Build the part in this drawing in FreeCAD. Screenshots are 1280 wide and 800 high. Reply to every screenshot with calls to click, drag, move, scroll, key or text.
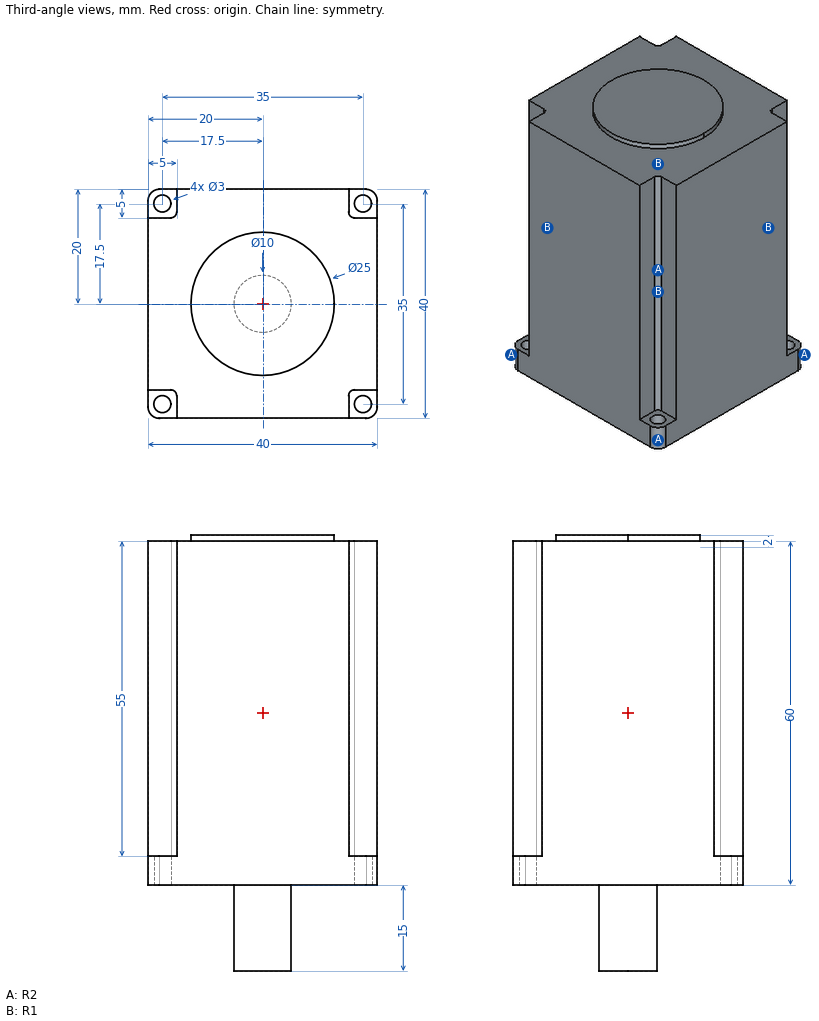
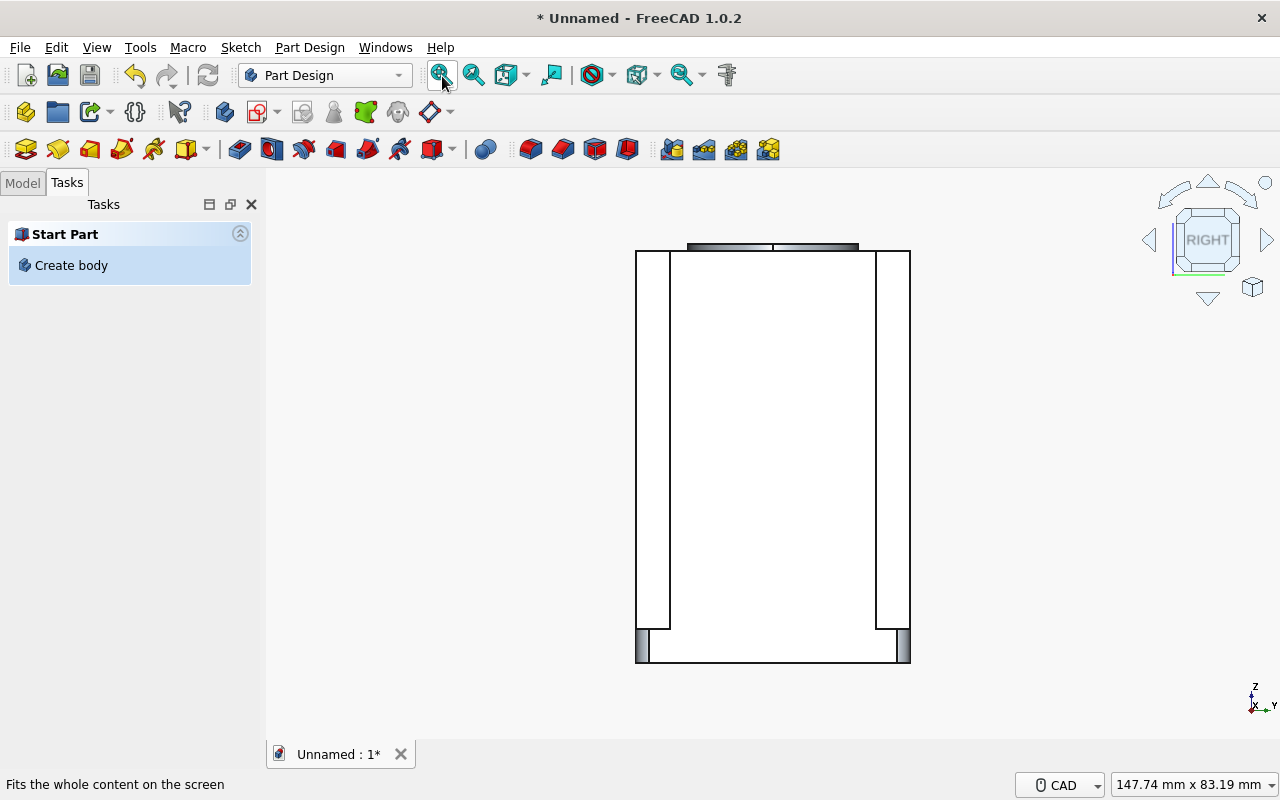
key(5)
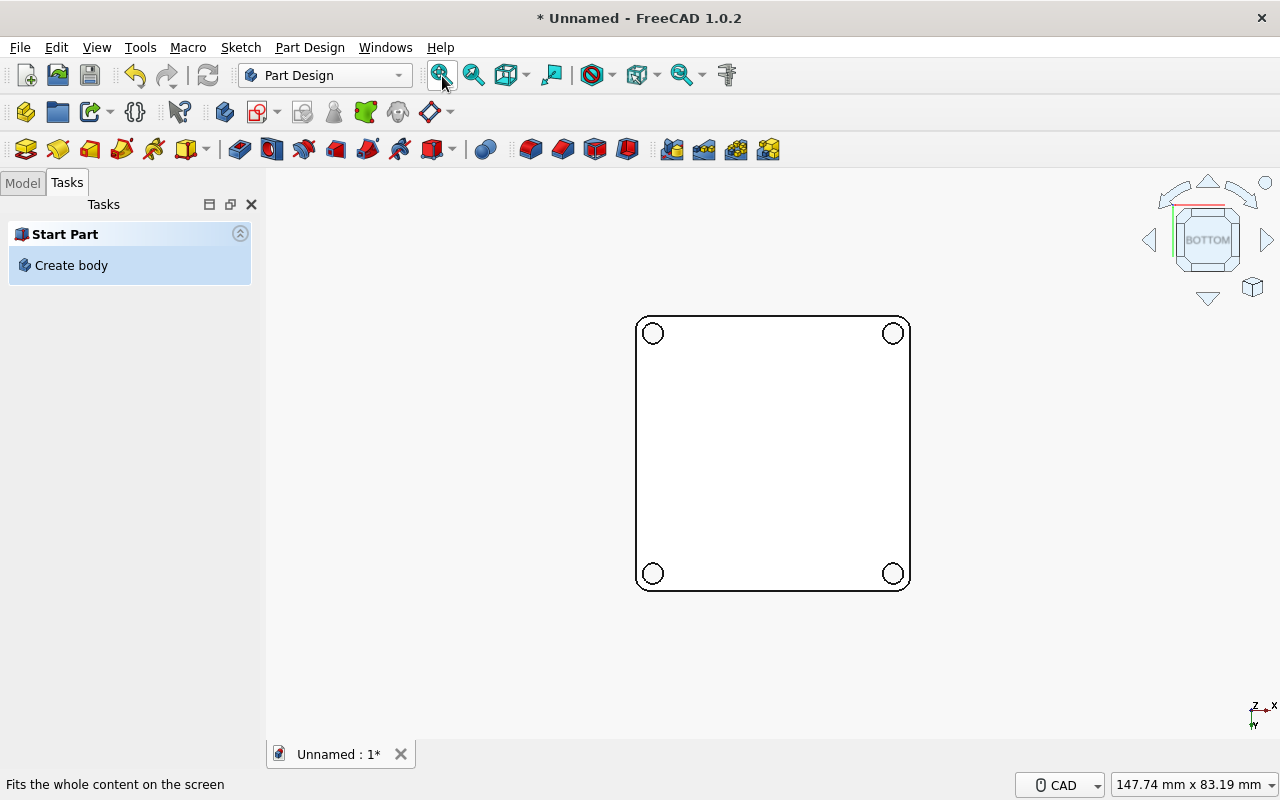
key(4)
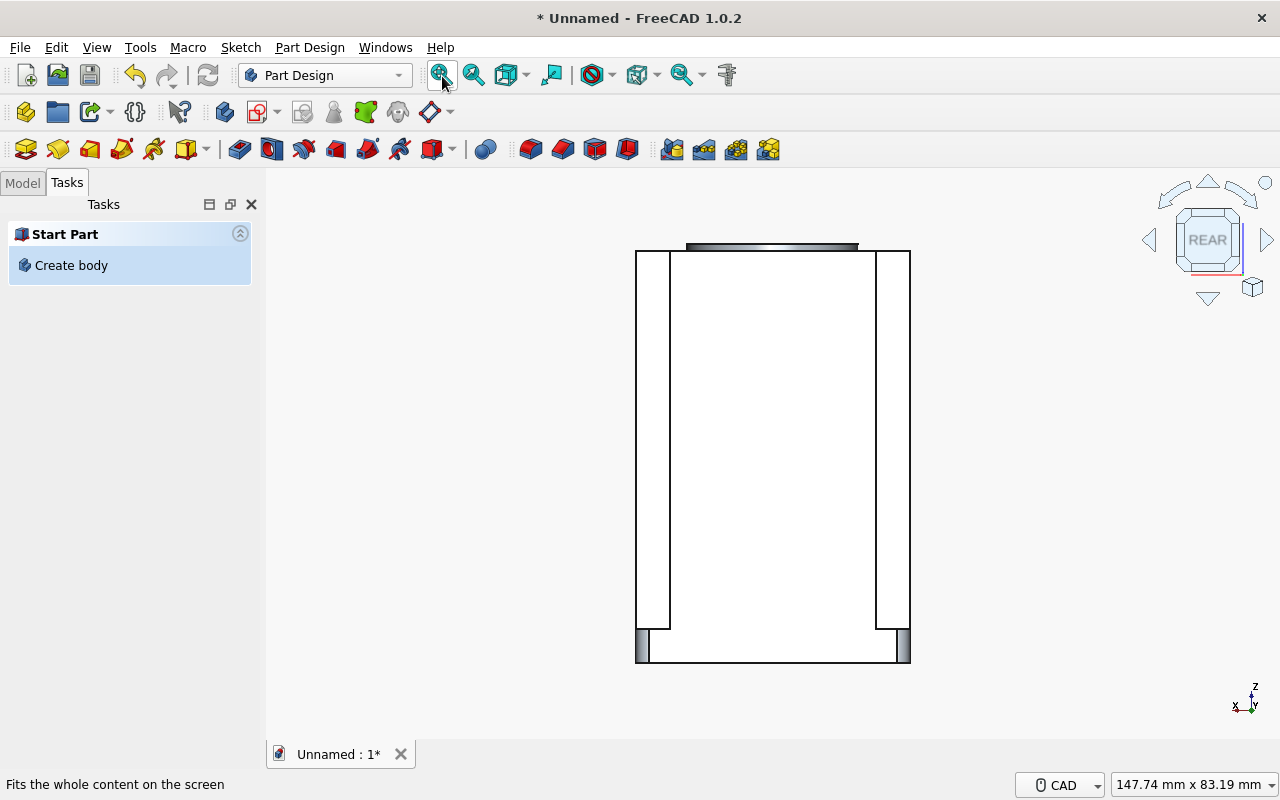
key(6)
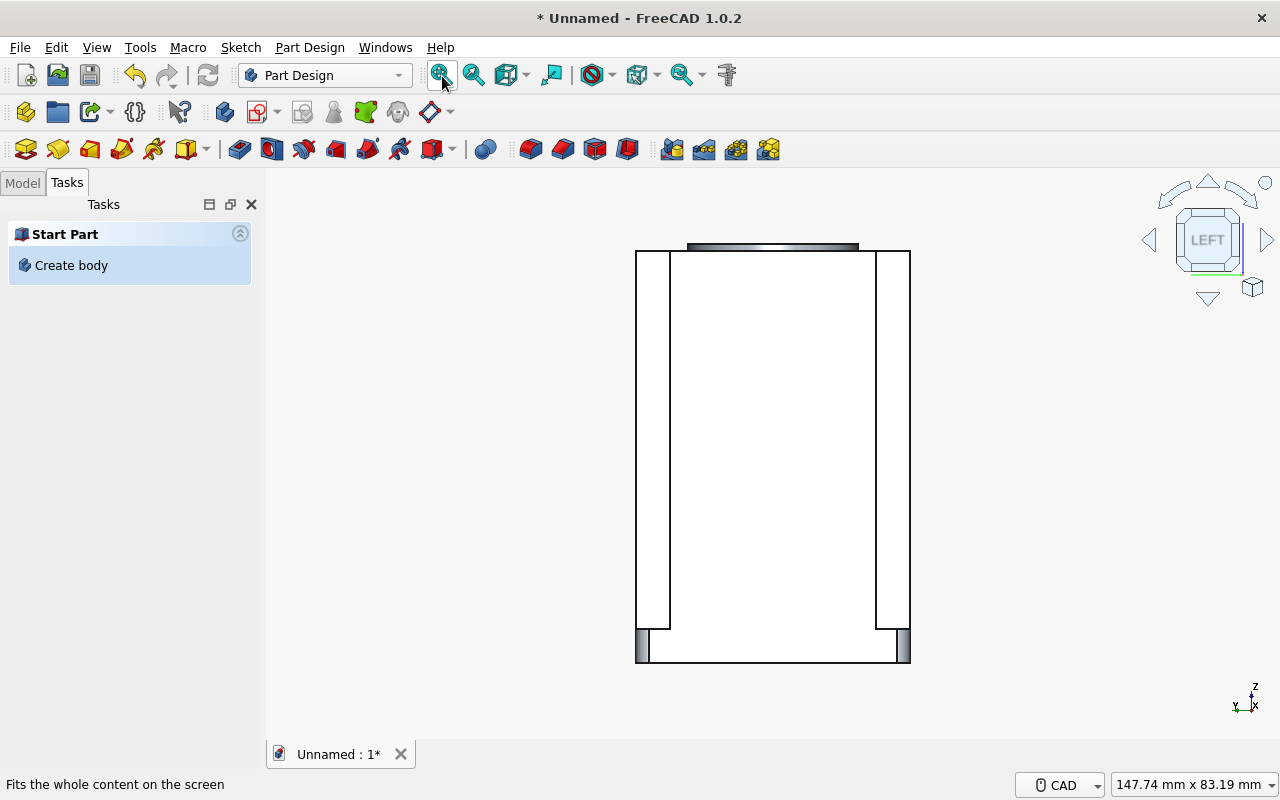
key(v)
key(3)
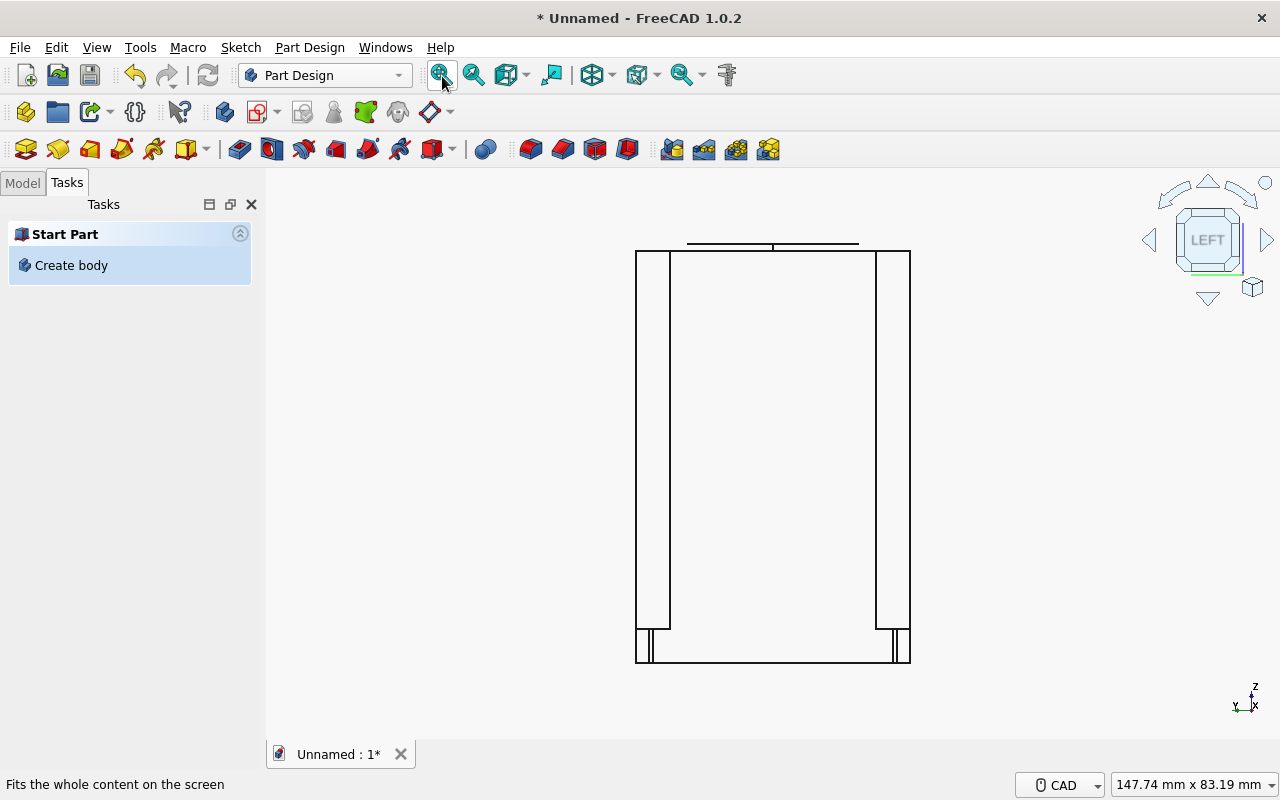
key(0)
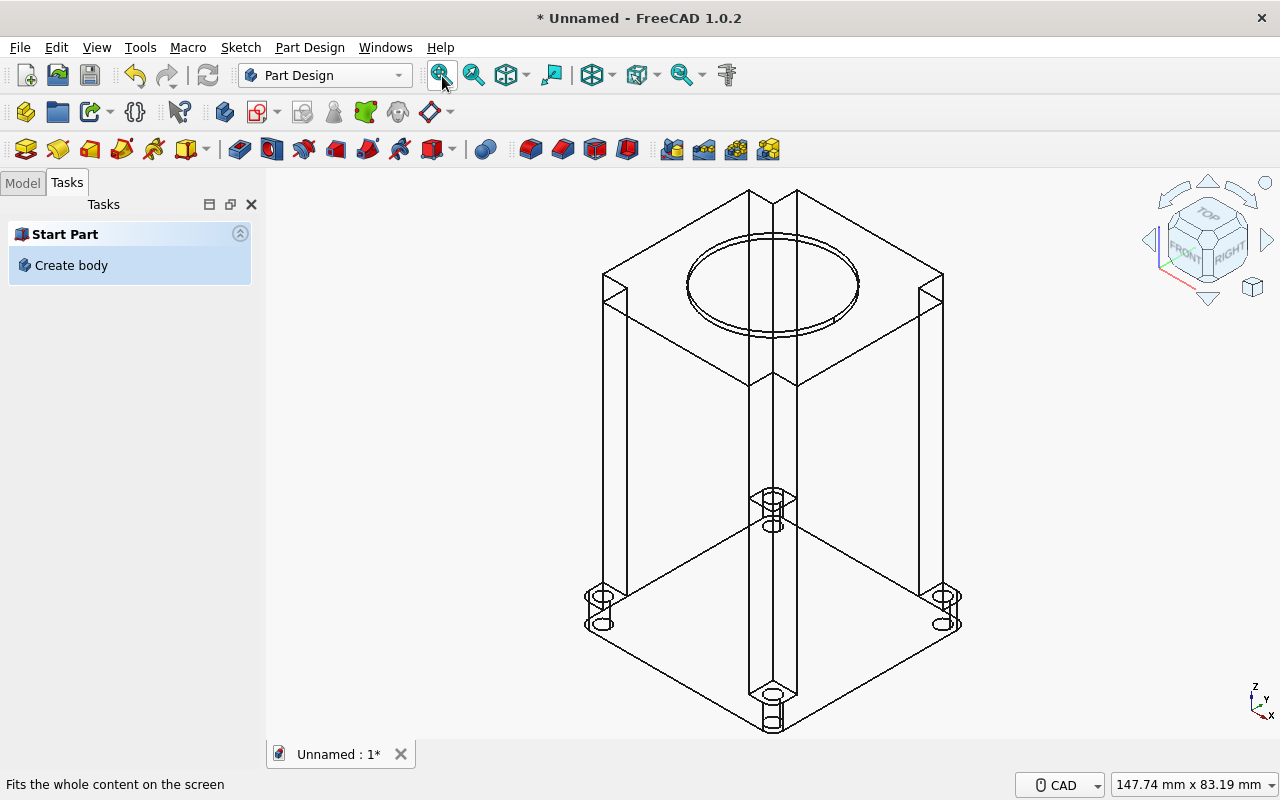
click(627, 441)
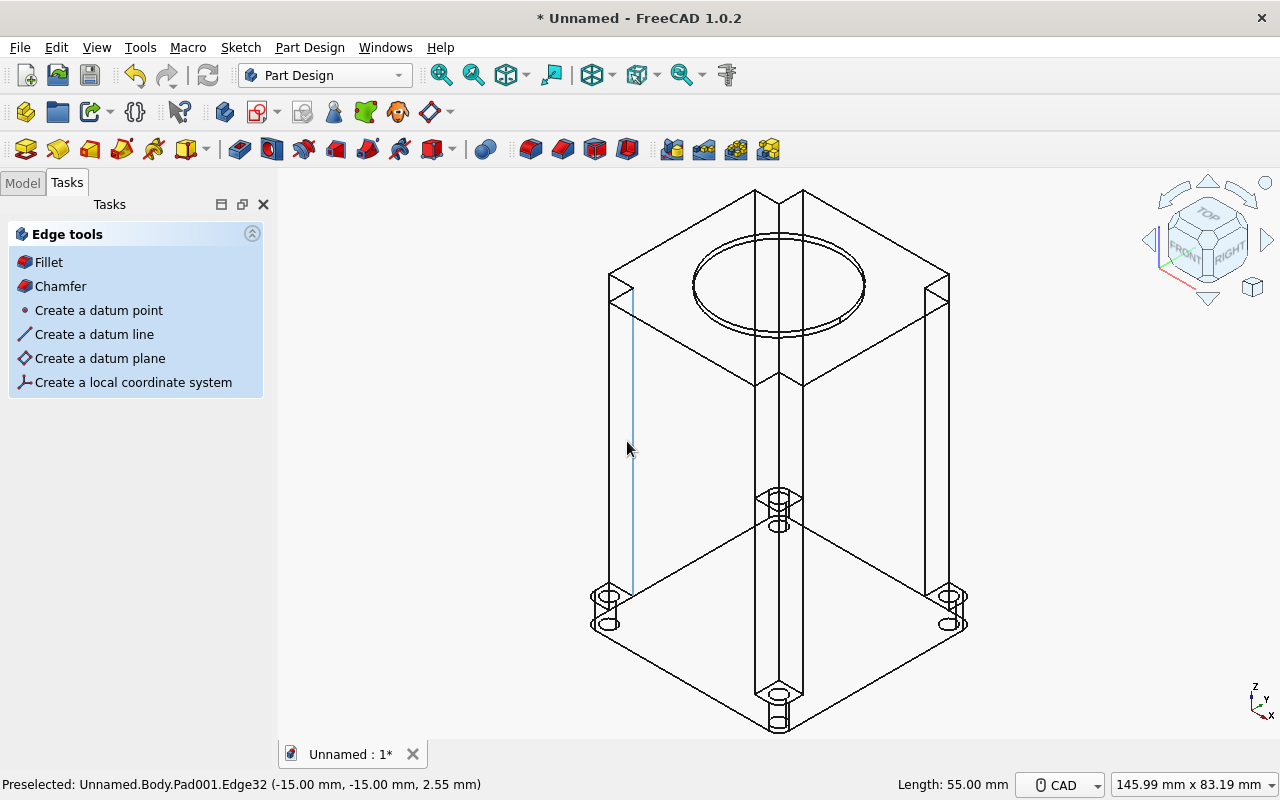
click(779, 525, ctrl)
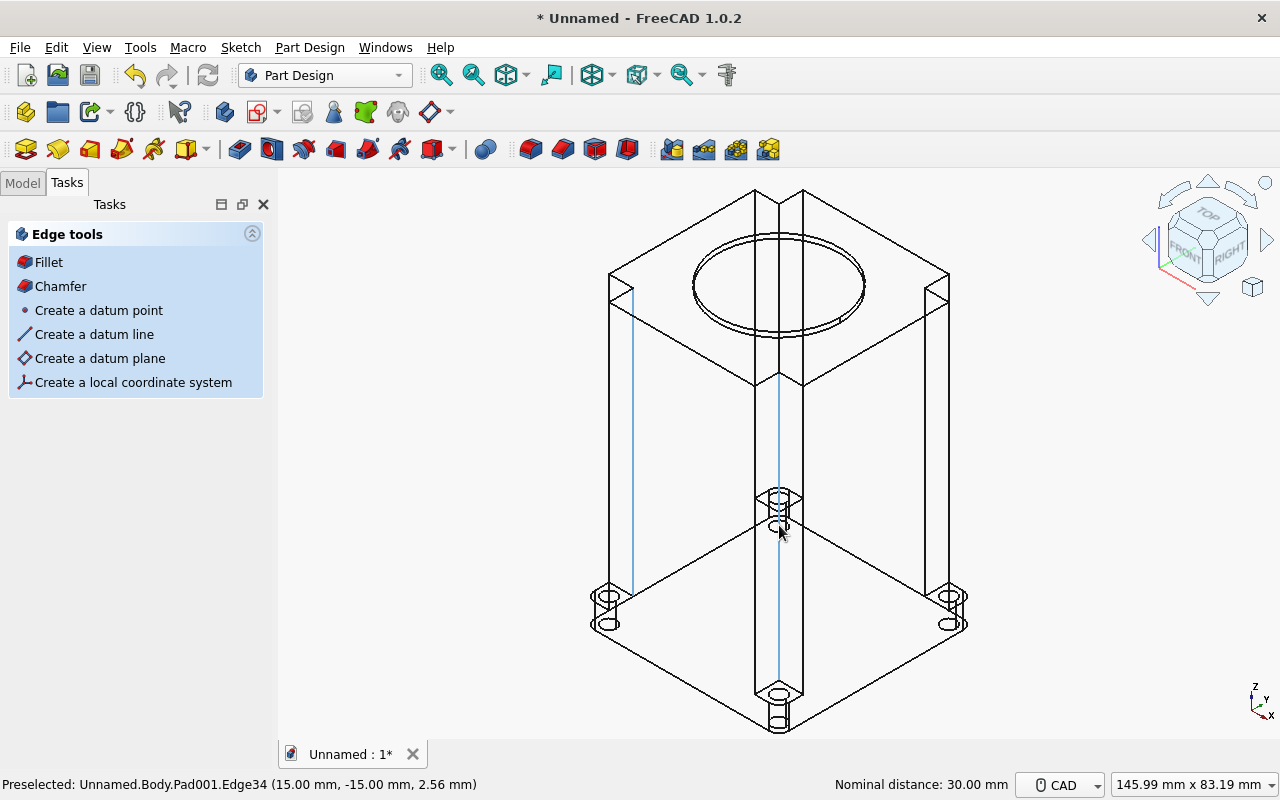
click(925, 441, ctrl)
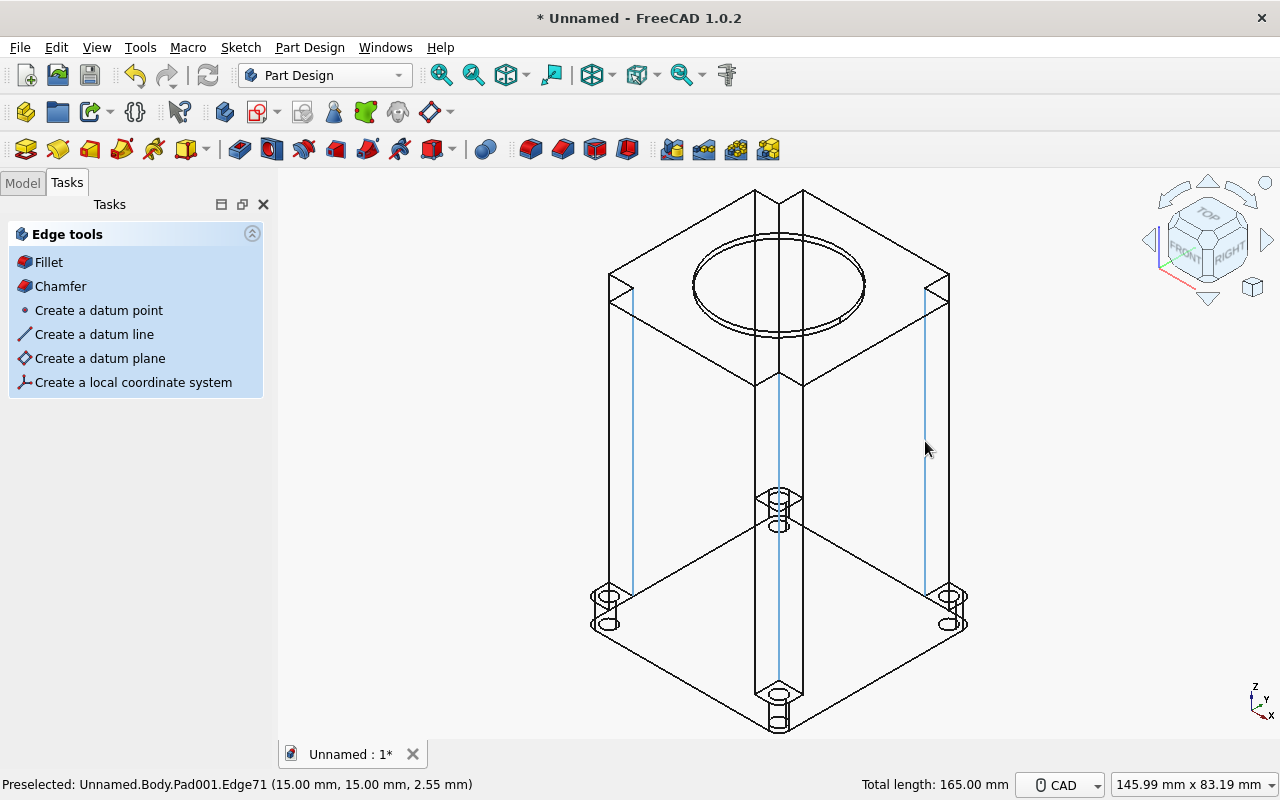
click(779, 357, ctrl)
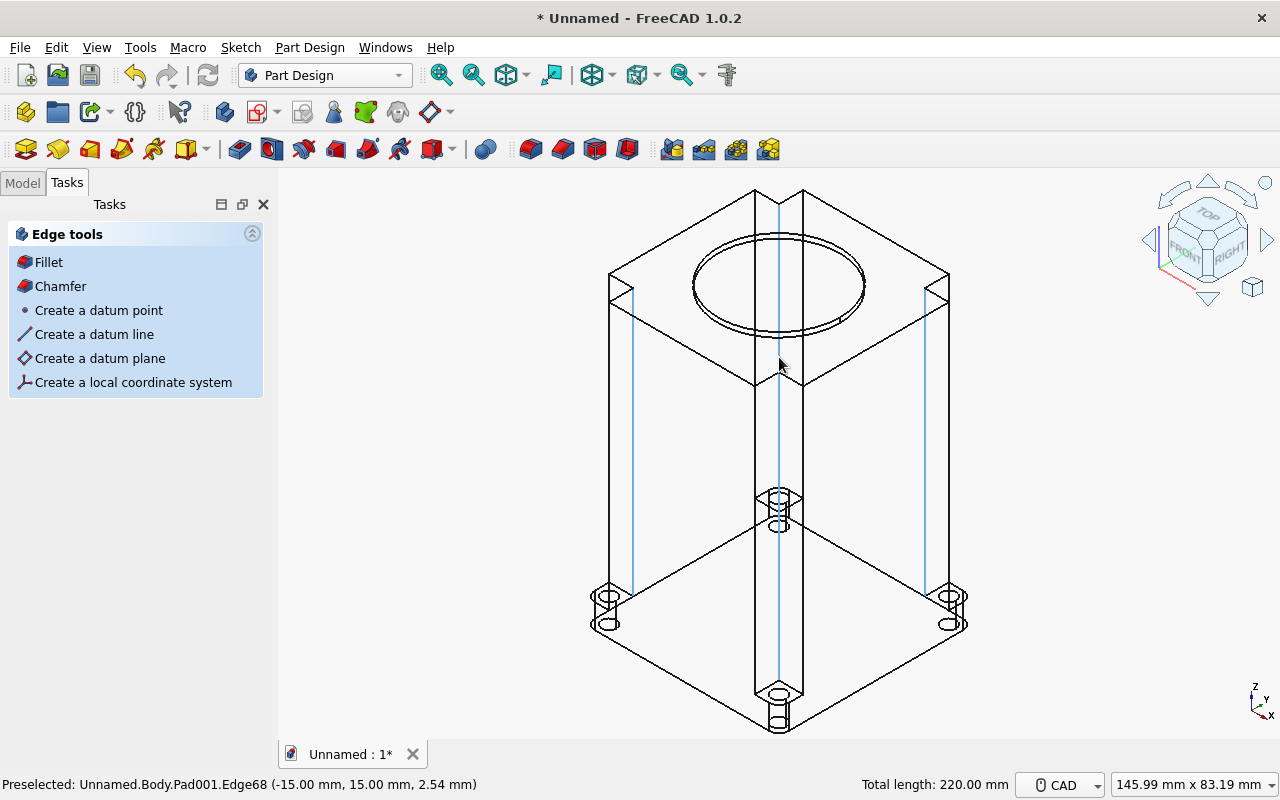
key(v)
key(1)